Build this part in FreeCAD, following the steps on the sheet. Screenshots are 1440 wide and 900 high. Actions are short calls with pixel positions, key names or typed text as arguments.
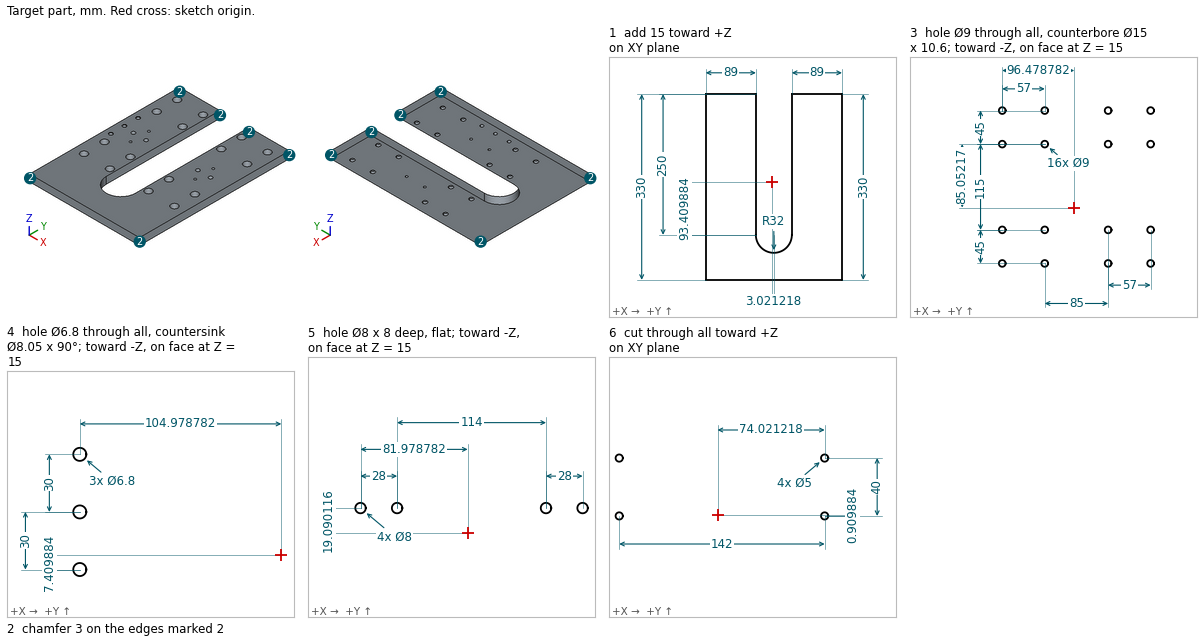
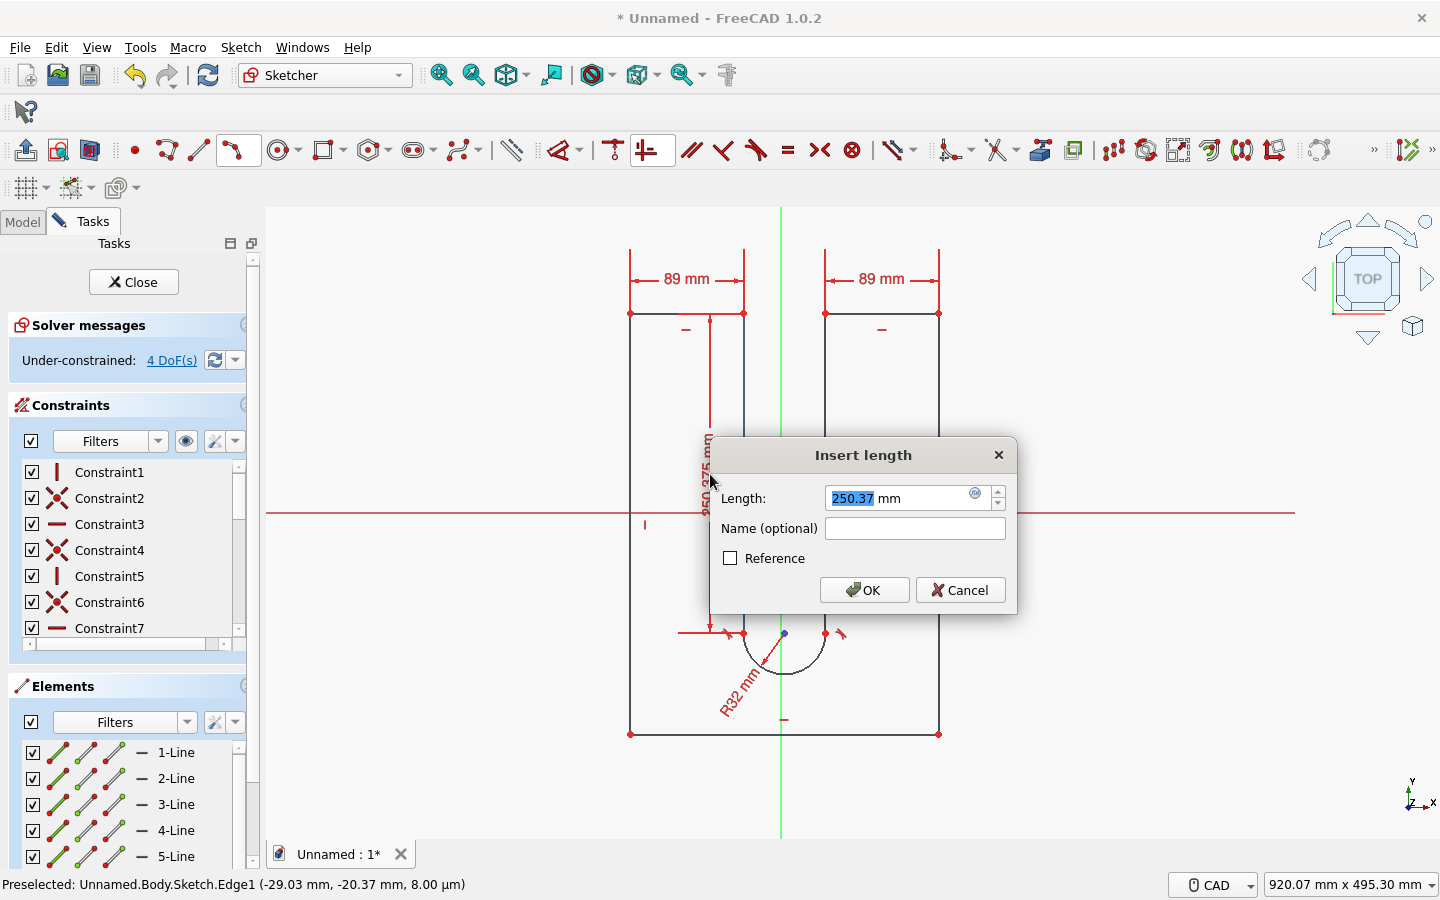
text(250)
key(Return)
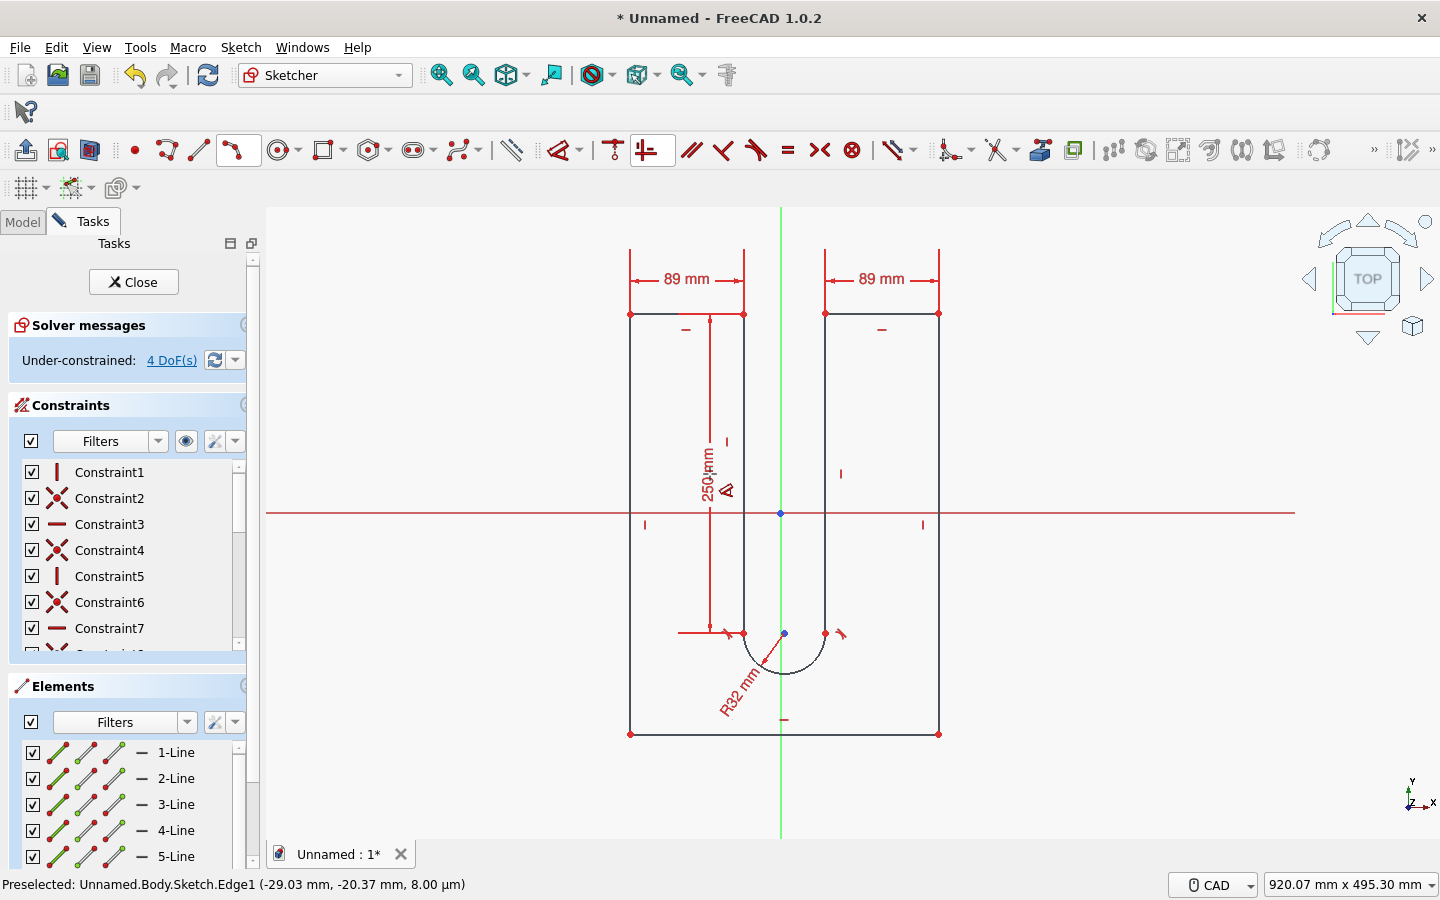
click(630, 440)
click(596, 428)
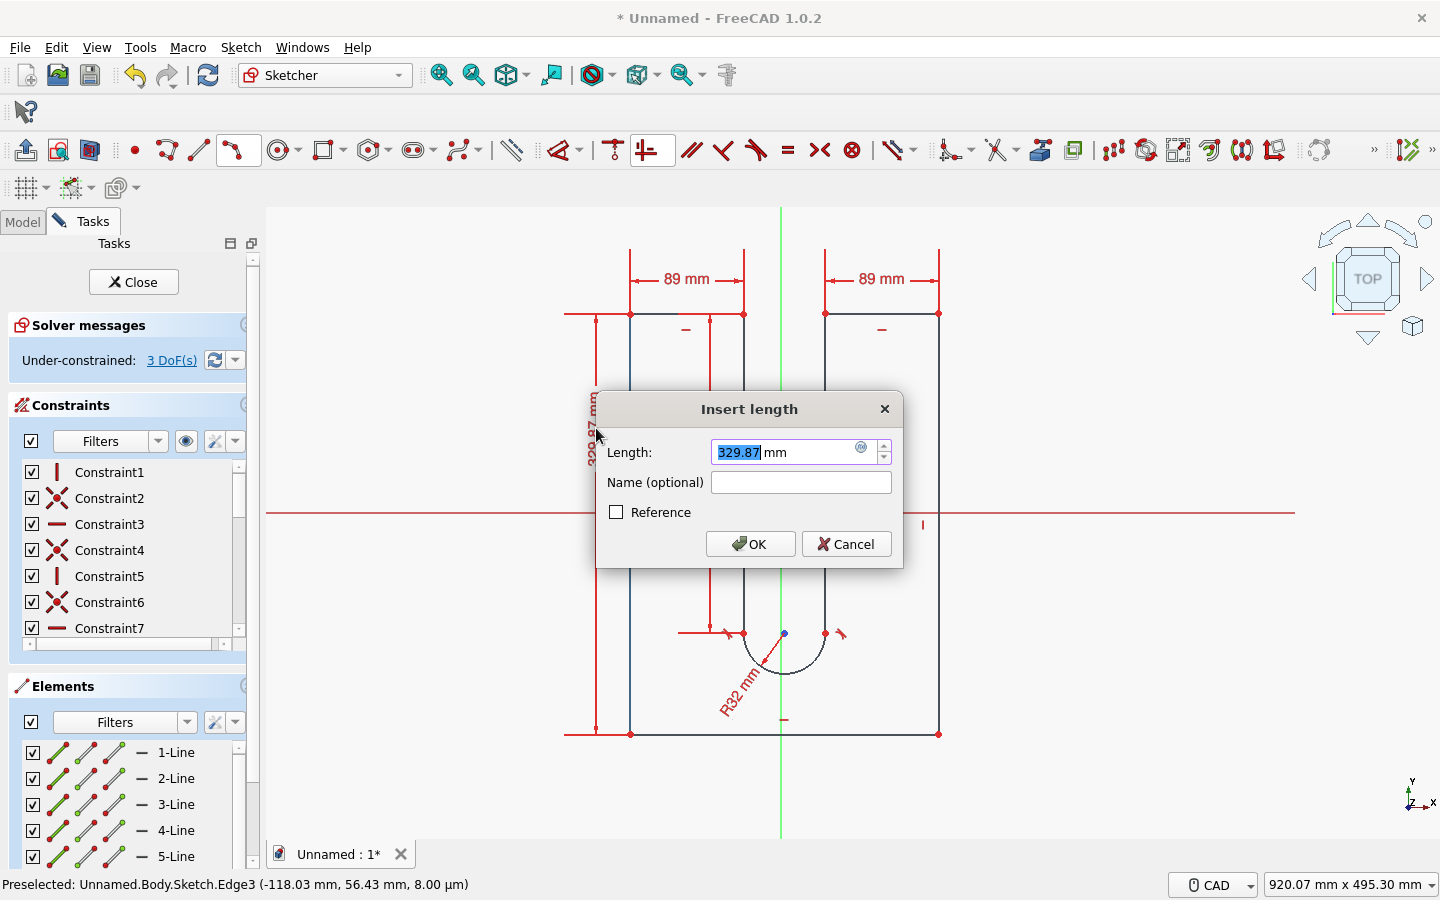
text(330)
key(Return)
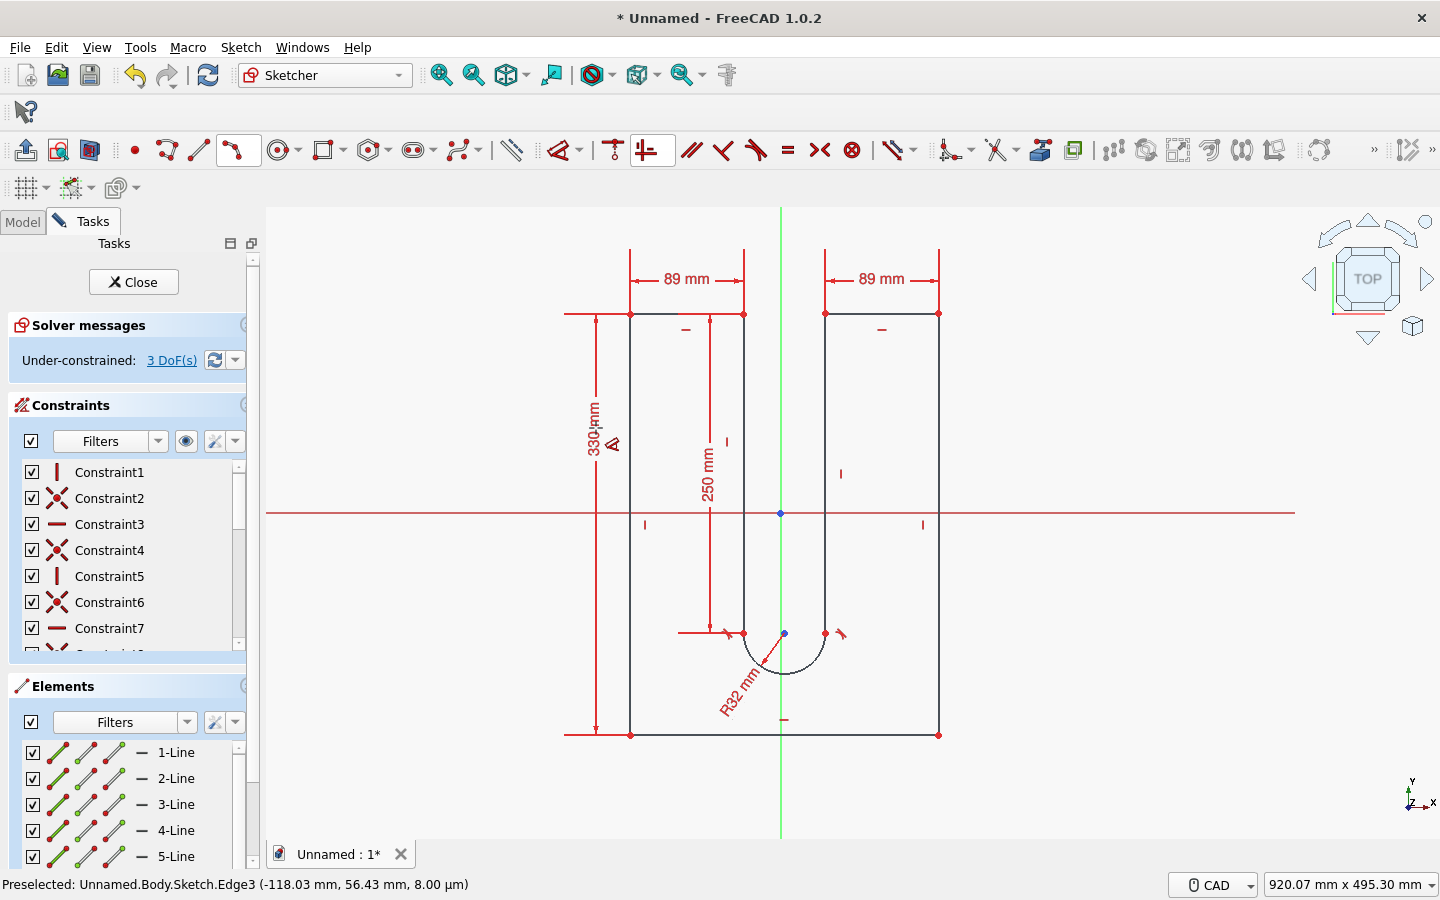
click(939, 609)
click(973, 428)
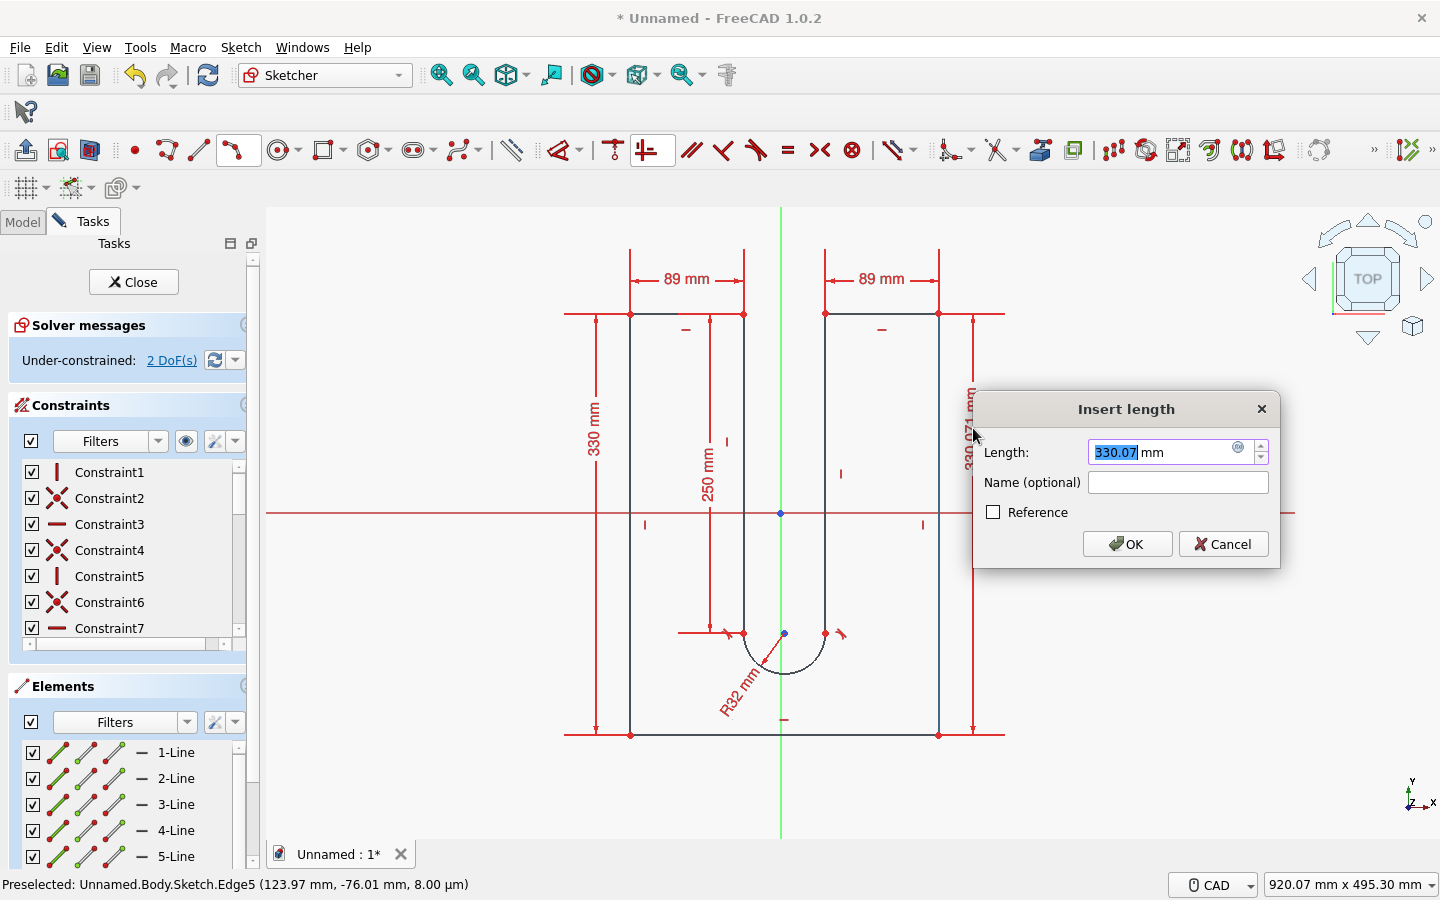
text(330)
key(Return)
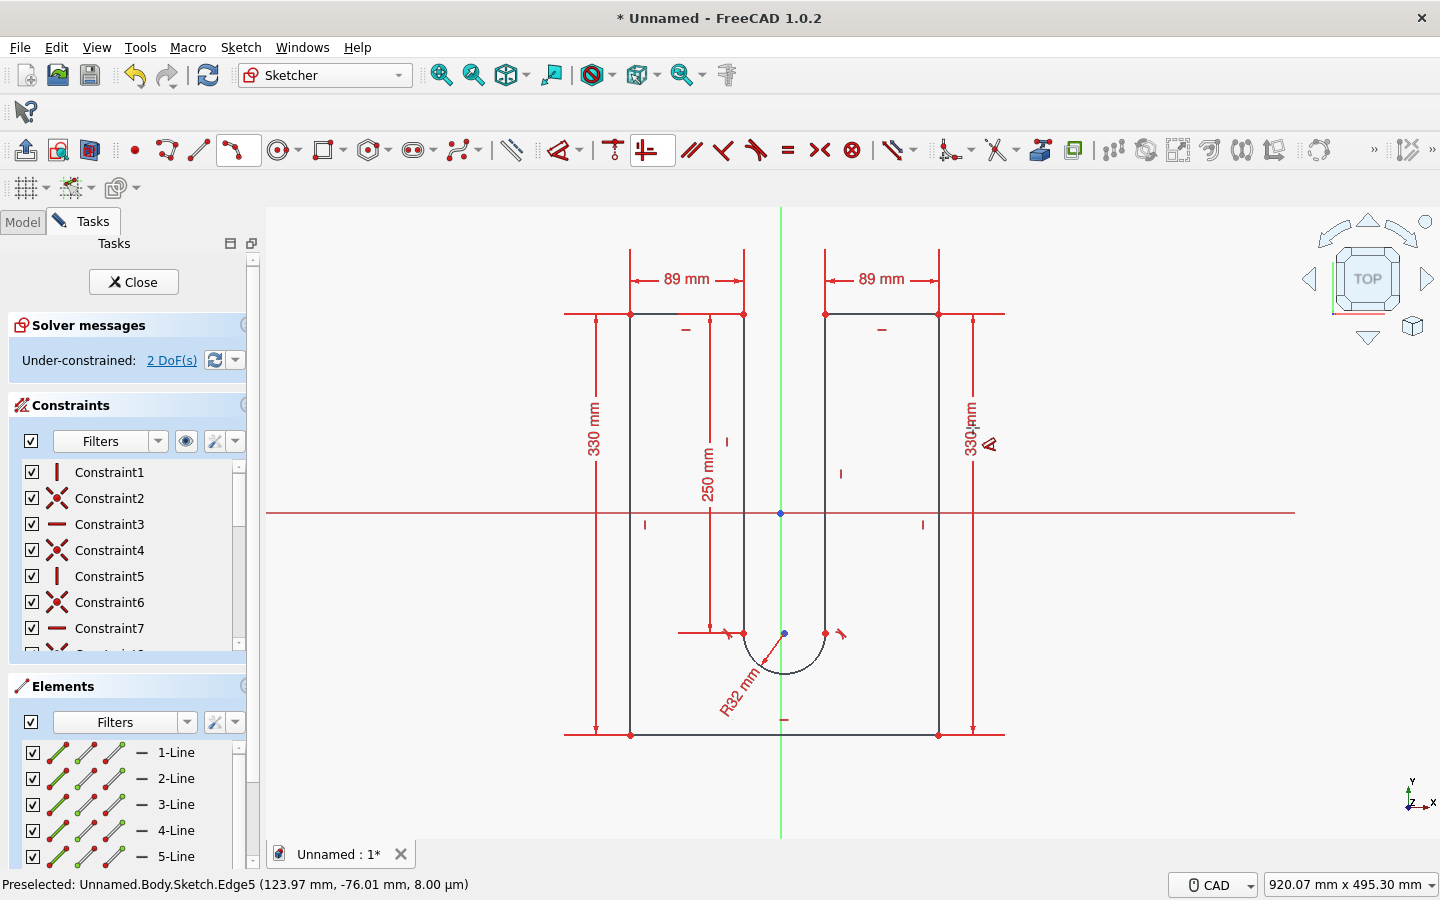
scroll(785, 633, up, 12)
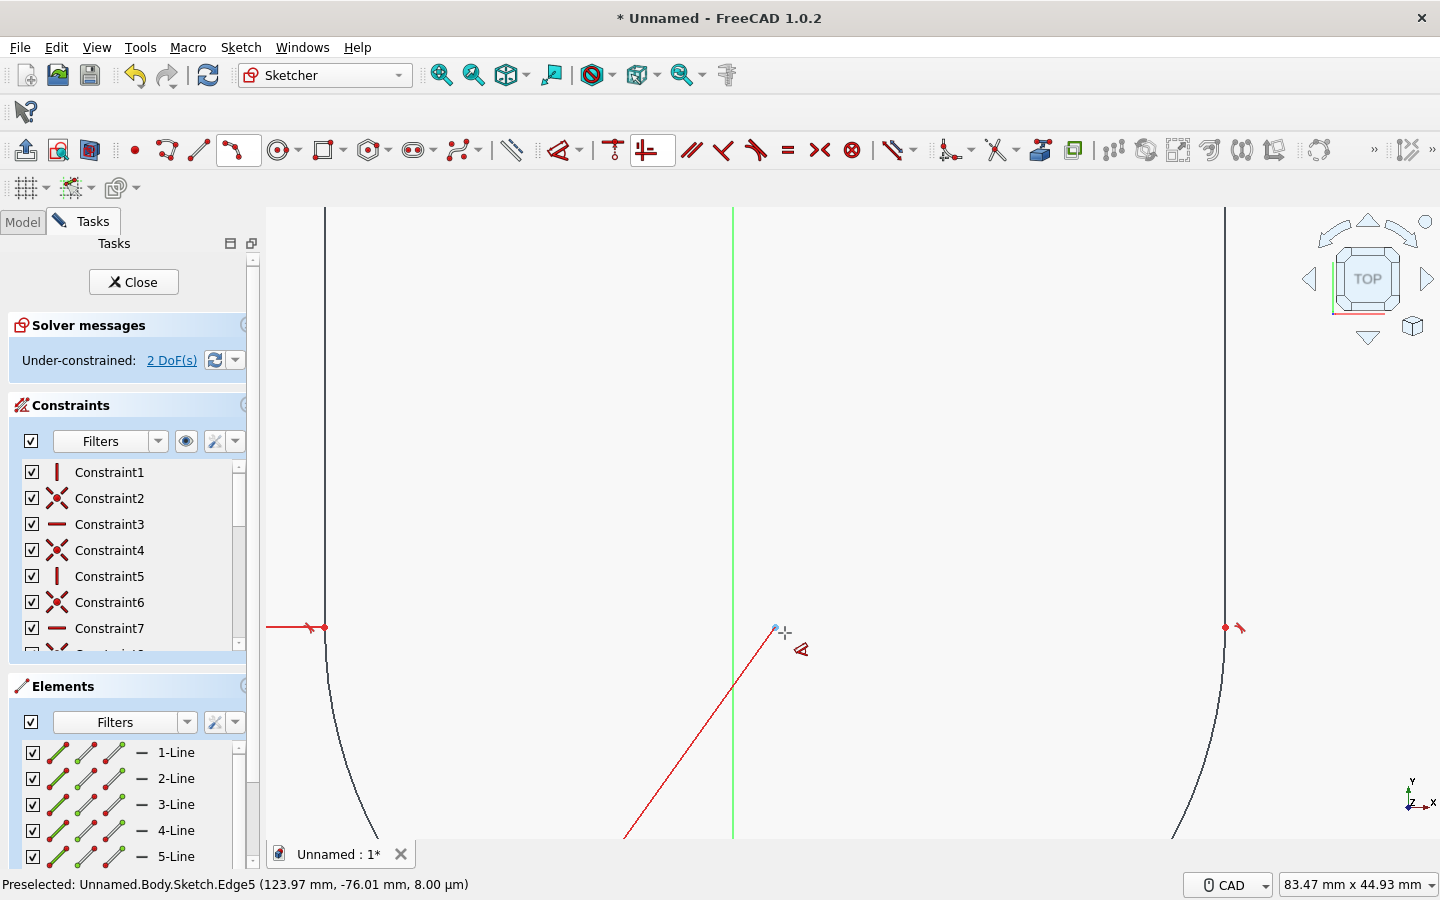
click(775, 627)
click(754, 661)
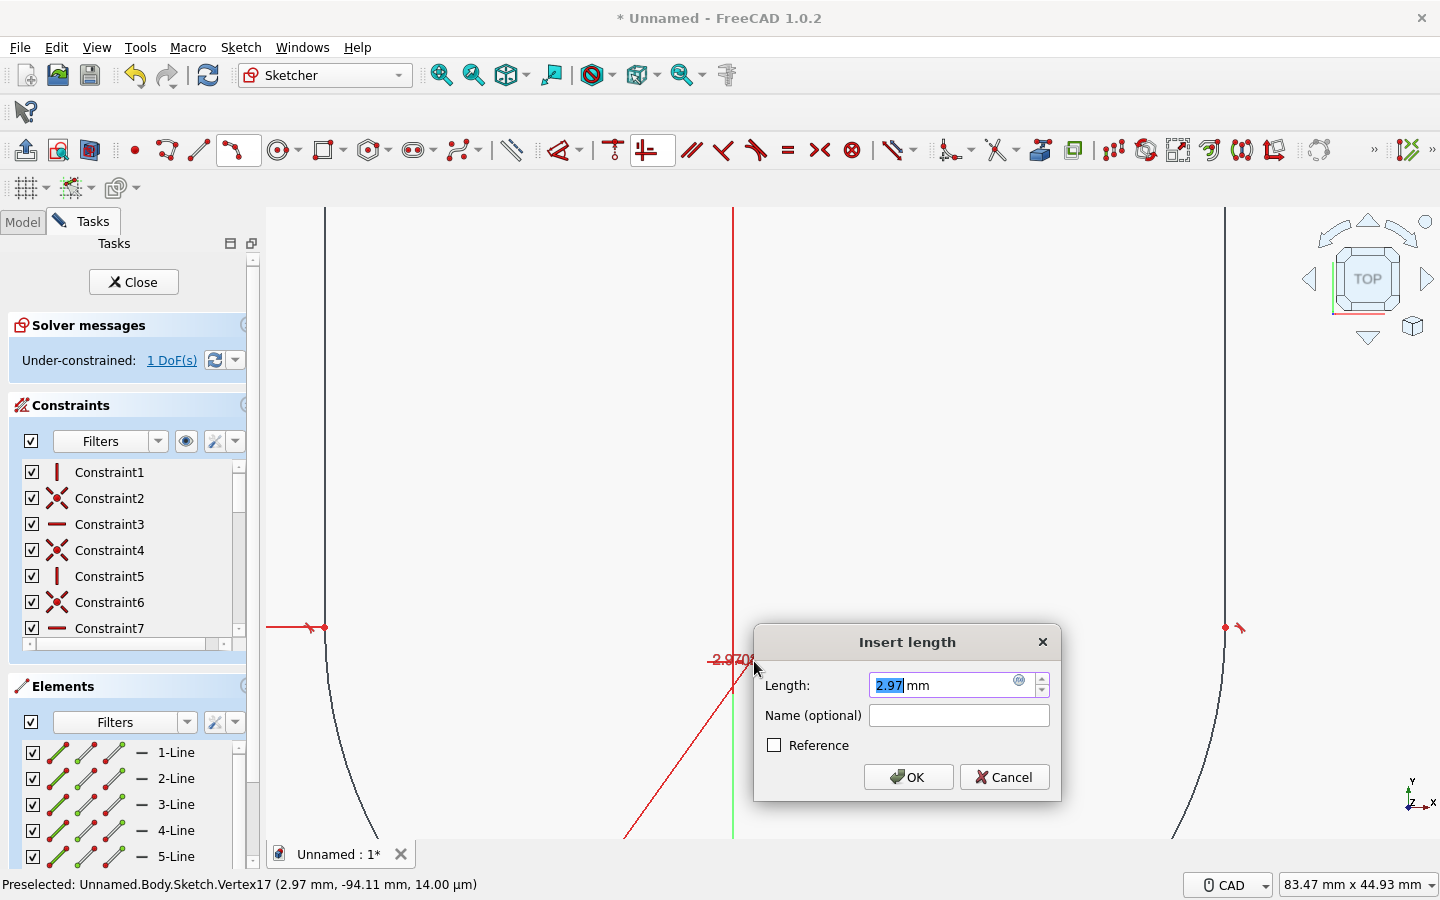
text(3.021218)
key(Return)